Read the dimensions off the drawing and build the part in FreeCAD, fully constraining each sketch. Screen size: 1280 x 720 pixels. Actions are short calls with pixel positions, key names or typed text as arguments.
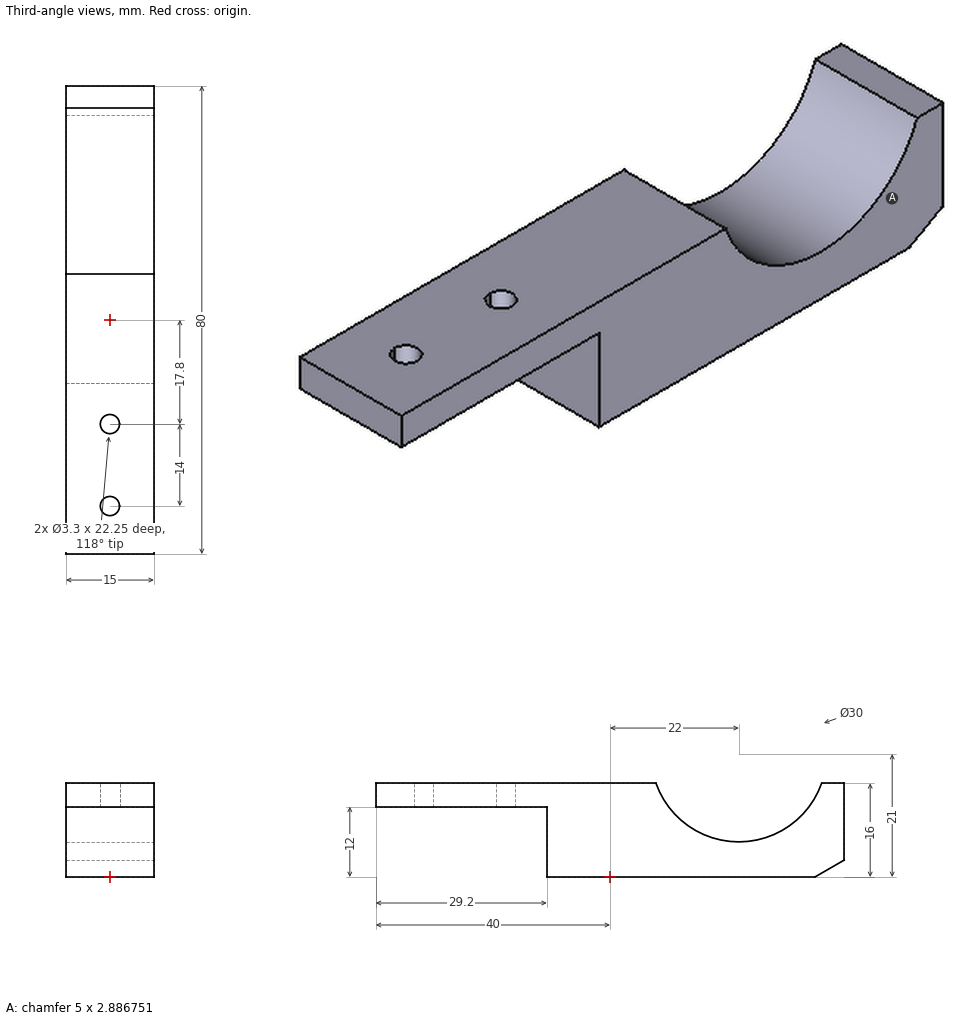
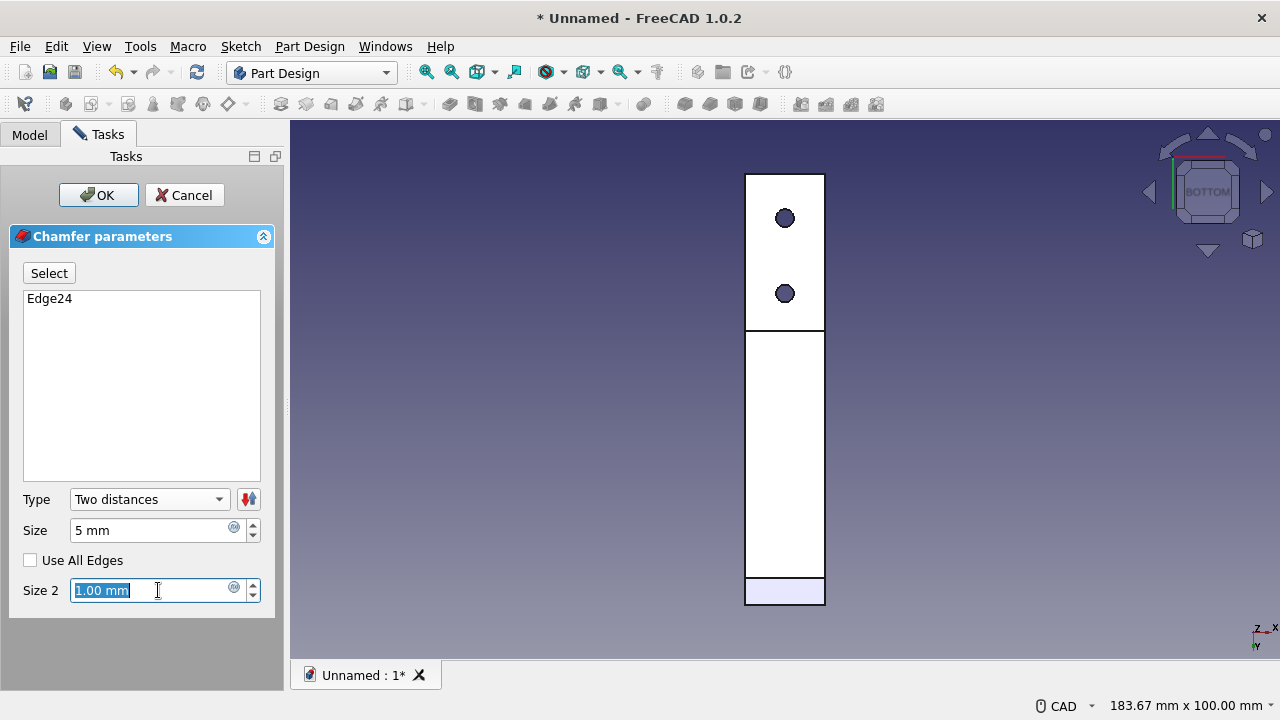
text(2.886751)
key(Tab)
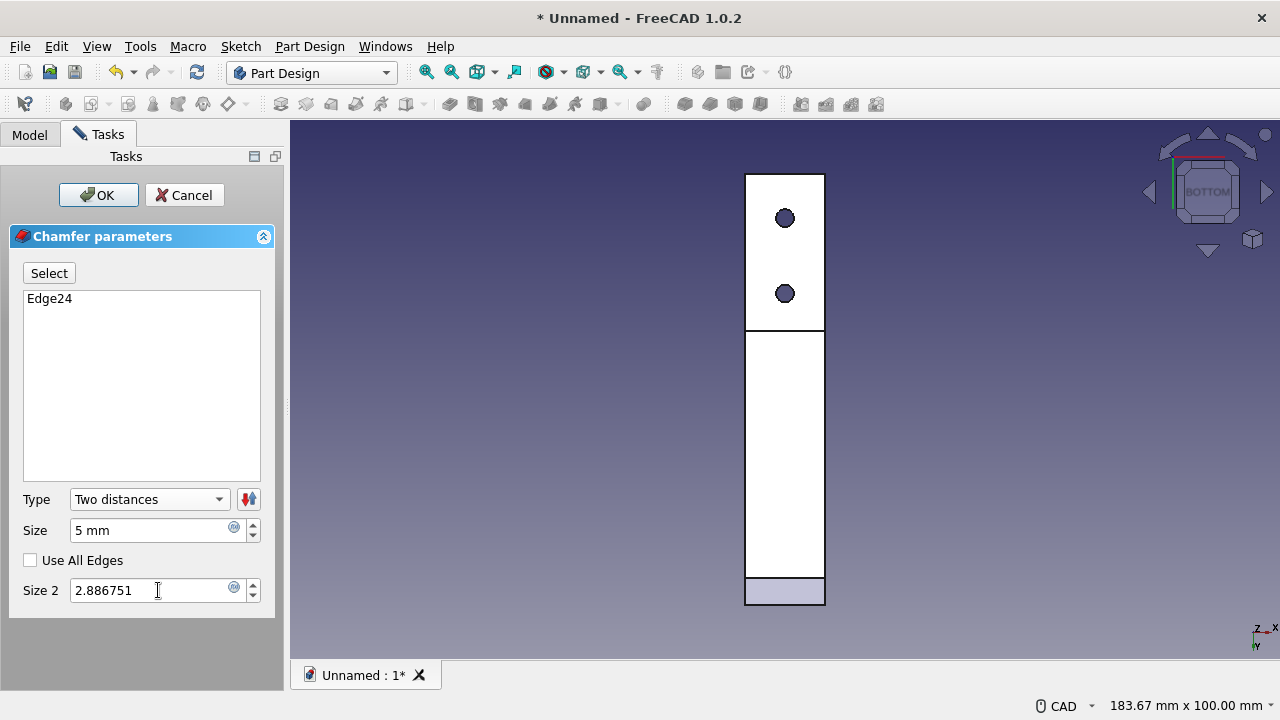
click(99, 195)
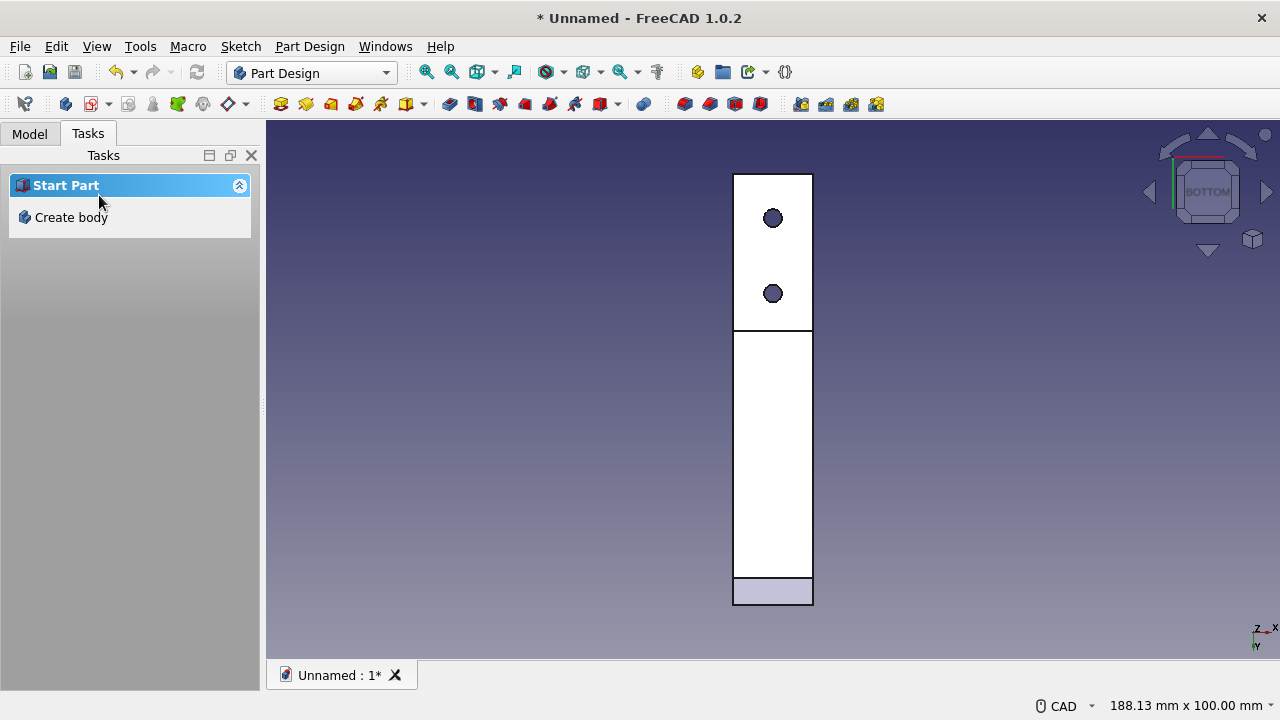
key(0)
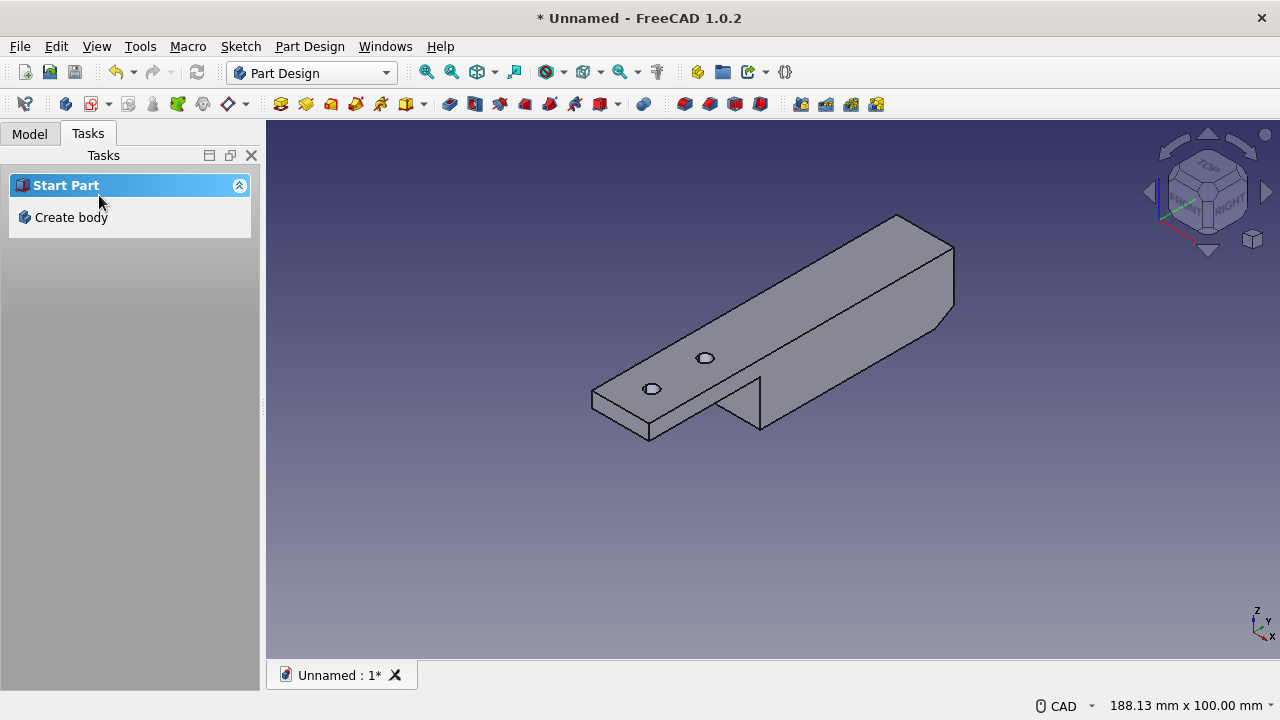
click(889, 319)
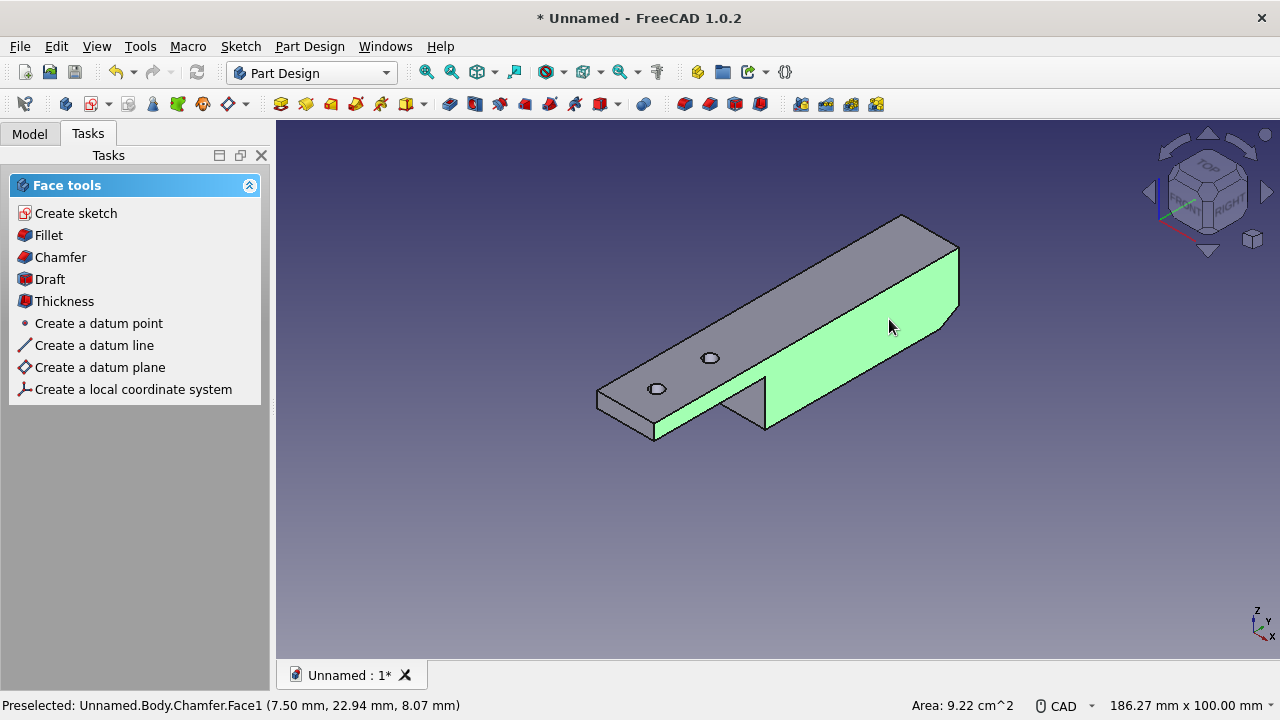
click(90, 104)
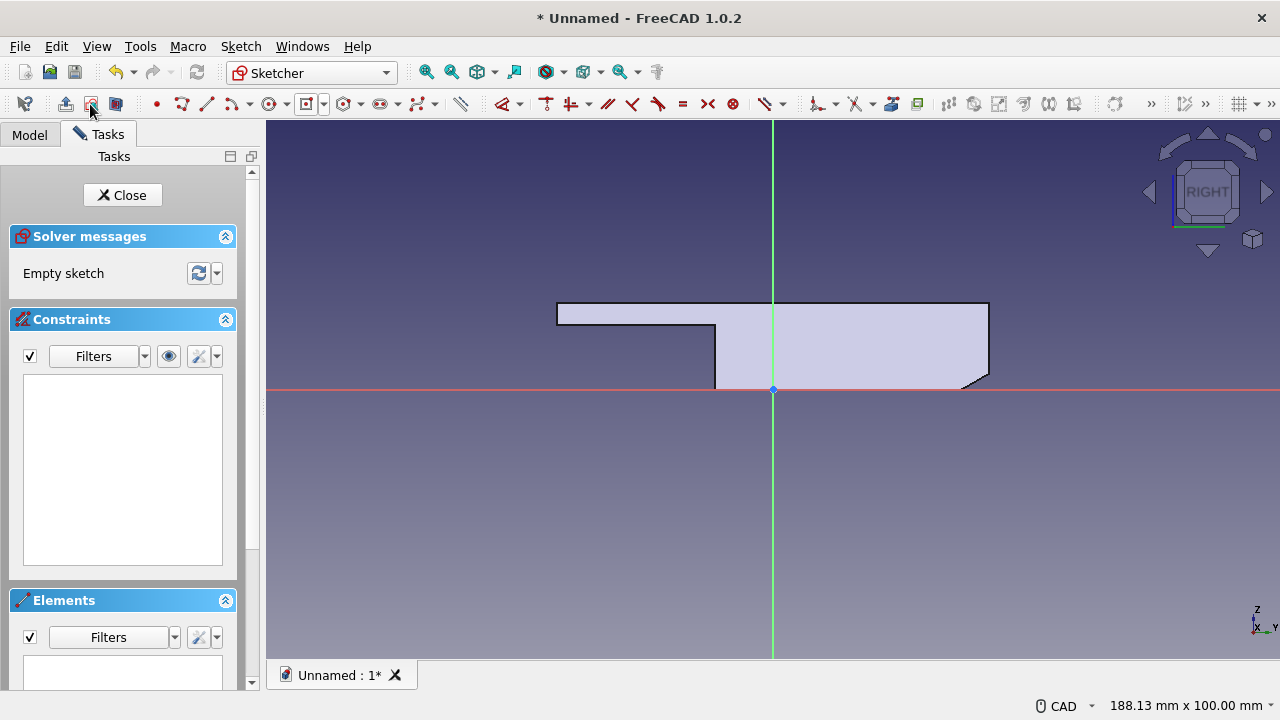
scroll(1077, 174, up, 3)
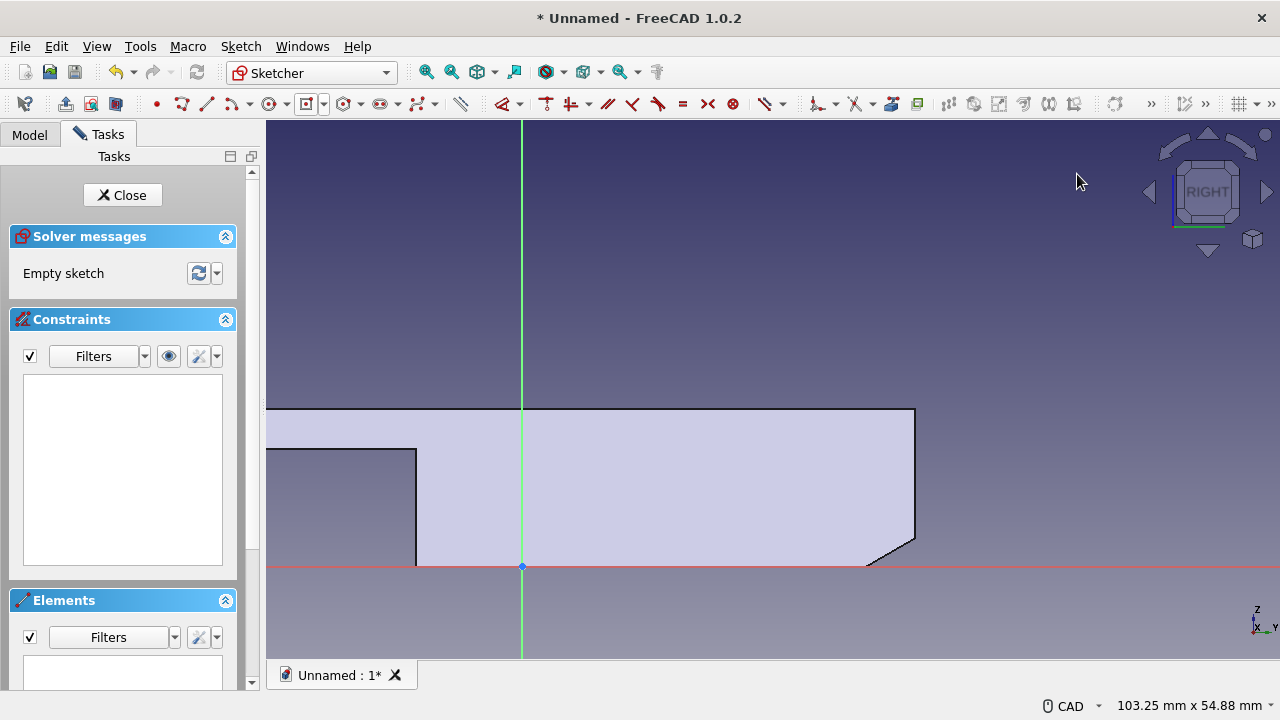
click(268, 104)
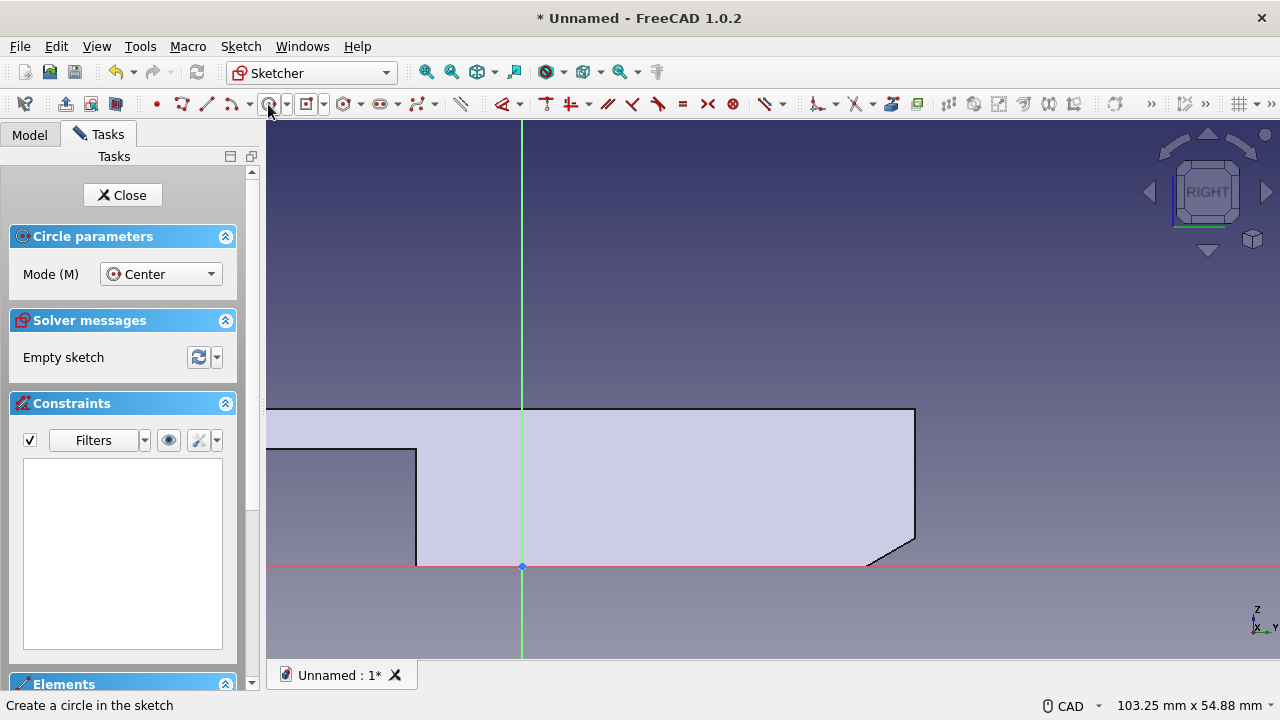
click(738, 360)
click(843, 256)
key(Escape)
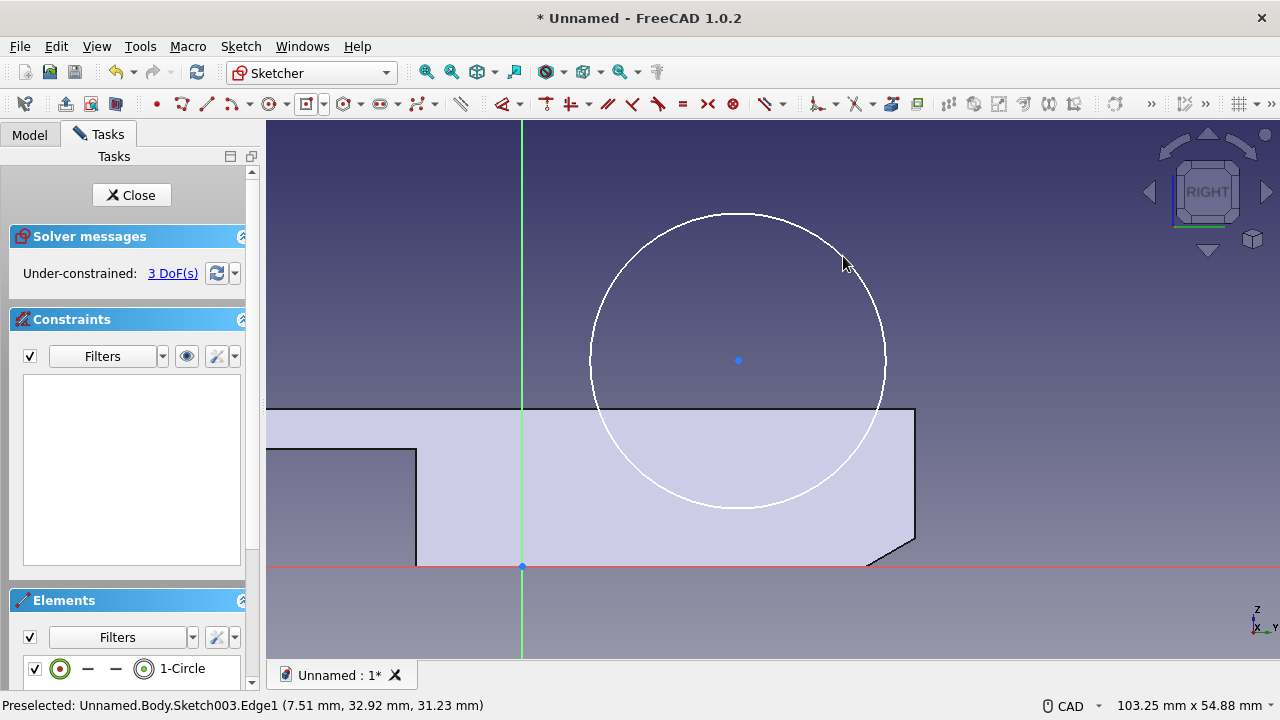
click(502, 104)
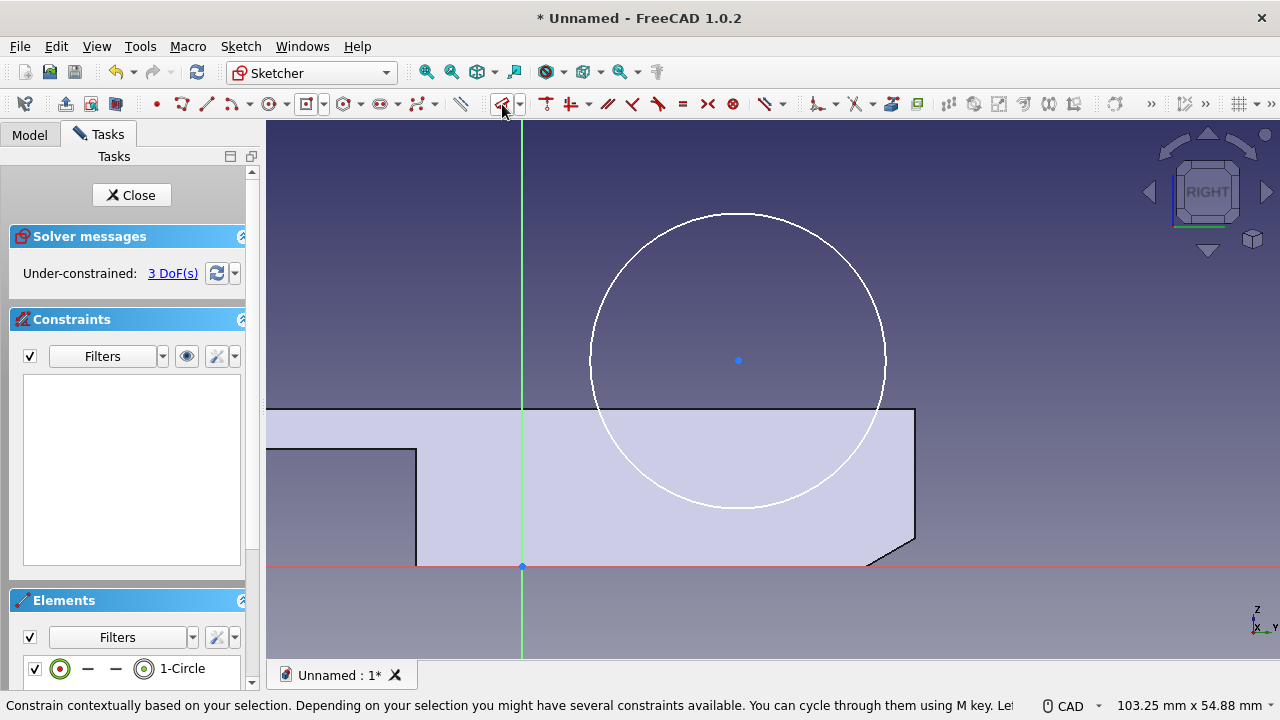
click(842, 256)
click(865, 233)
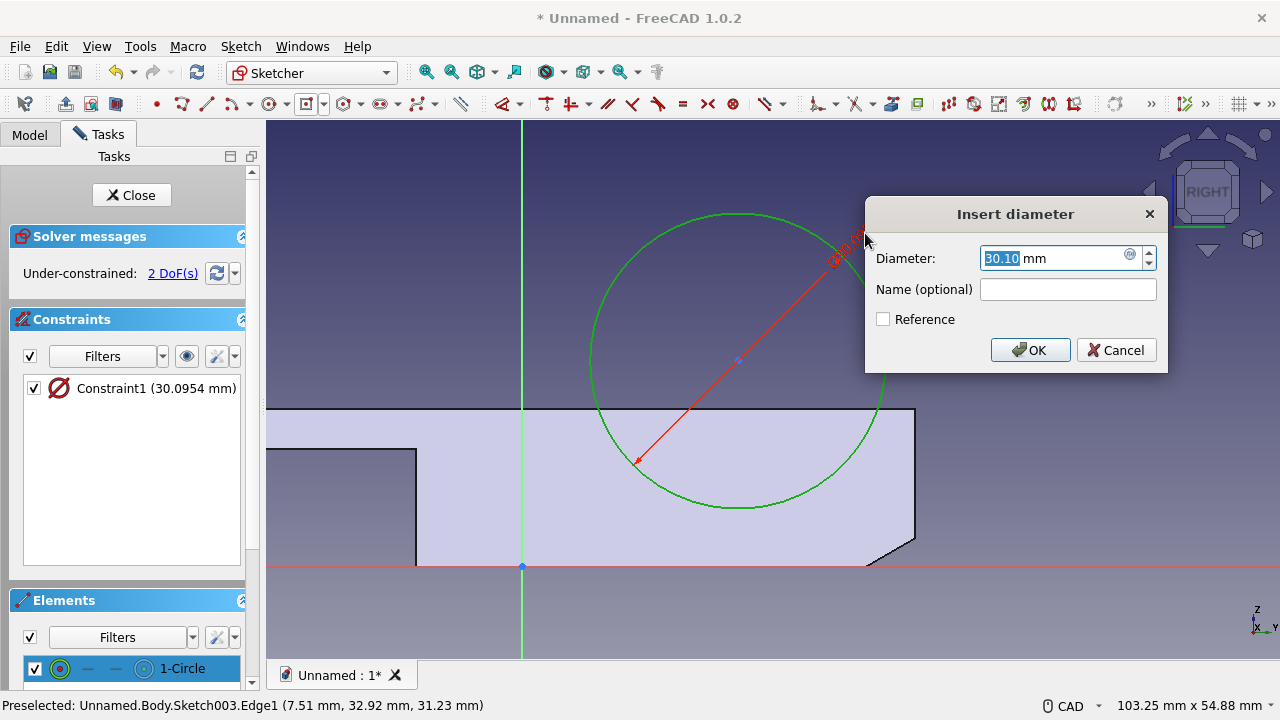
text(30)
key(Return)